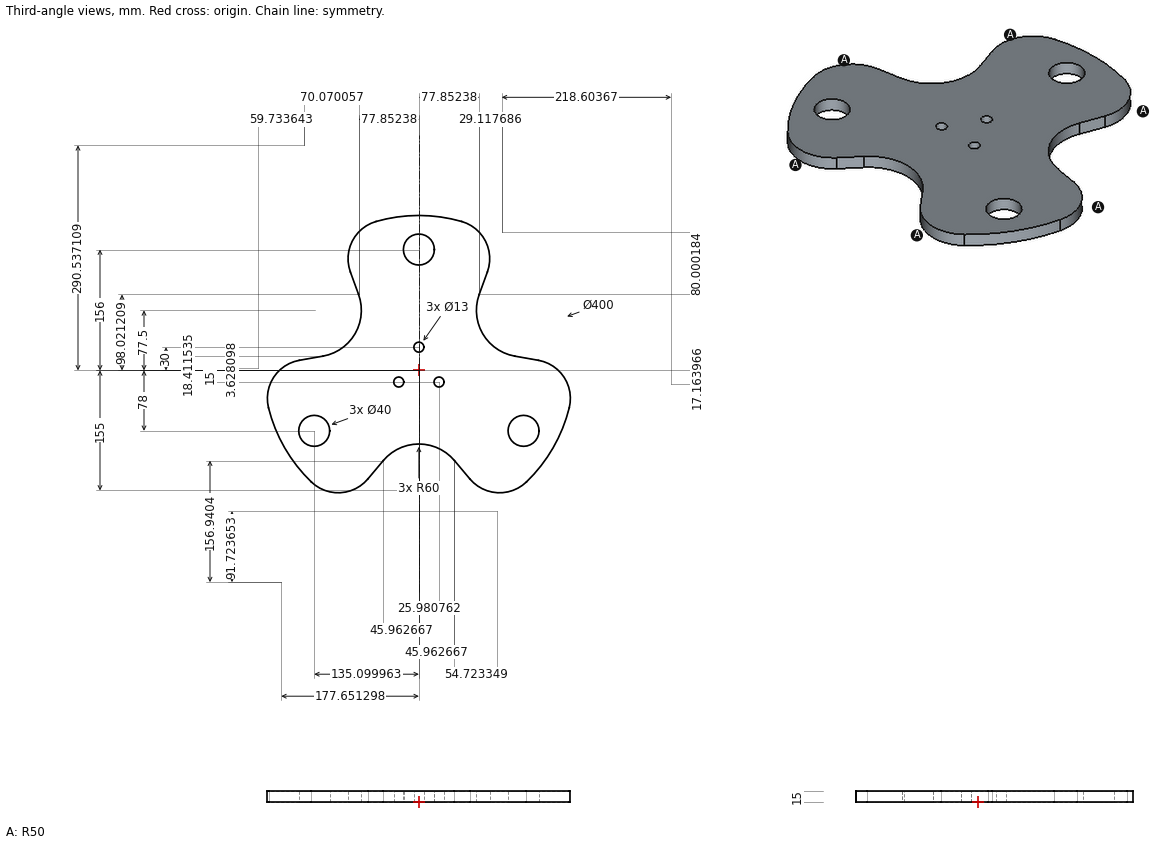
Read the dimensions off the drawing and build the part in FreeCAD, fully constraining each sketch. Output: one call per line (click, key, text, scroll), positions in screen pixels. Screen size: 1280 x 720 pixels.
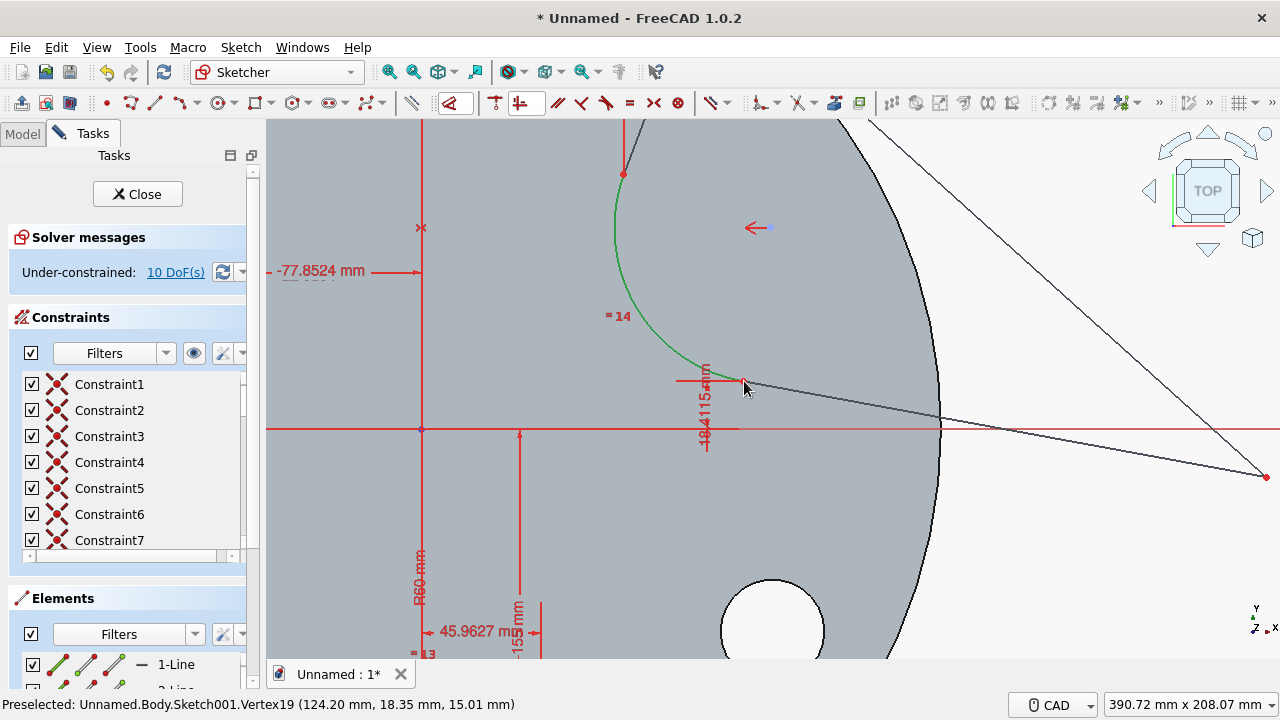
scroll(747, 383, down, 7)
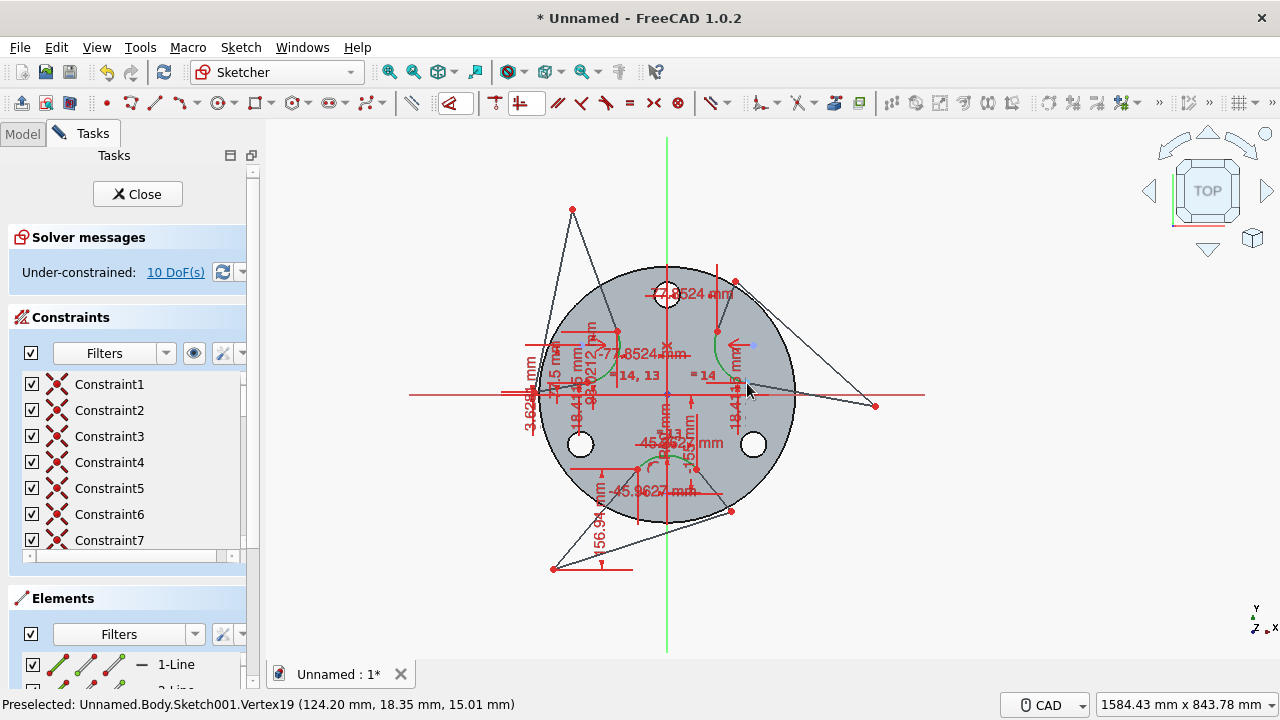
scroll(875, 407, up, 7)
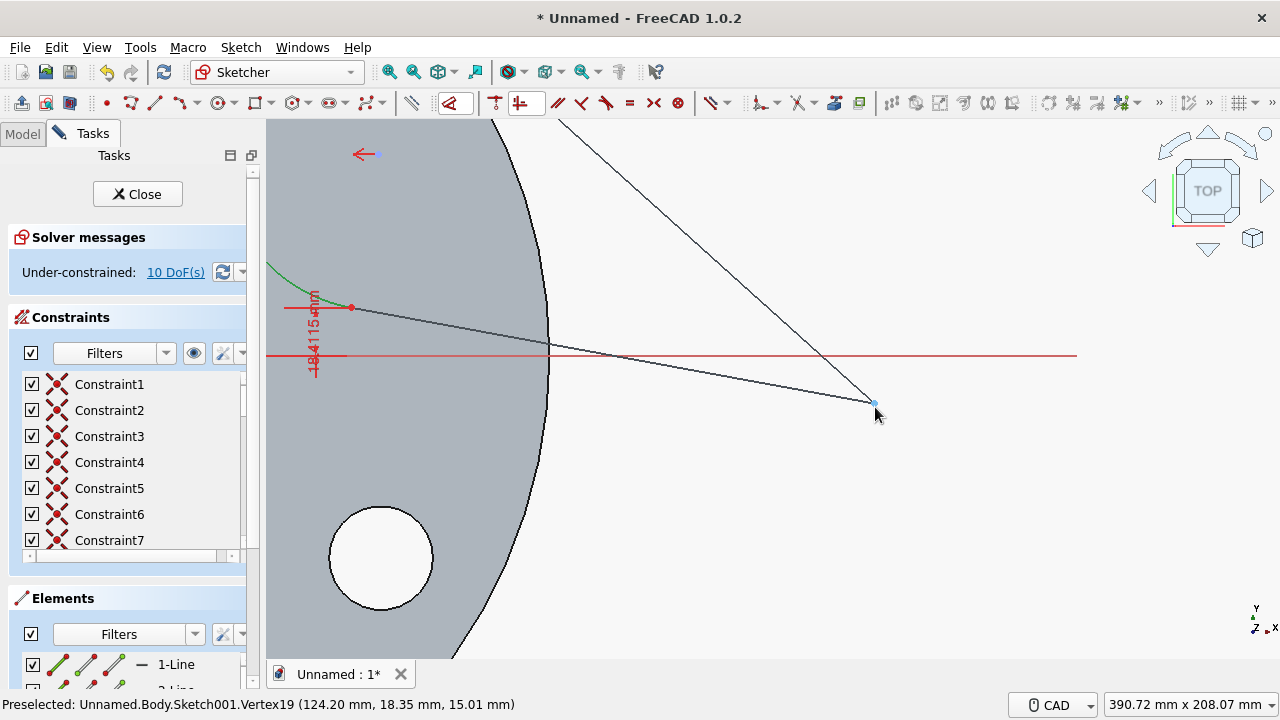
click(875, 404)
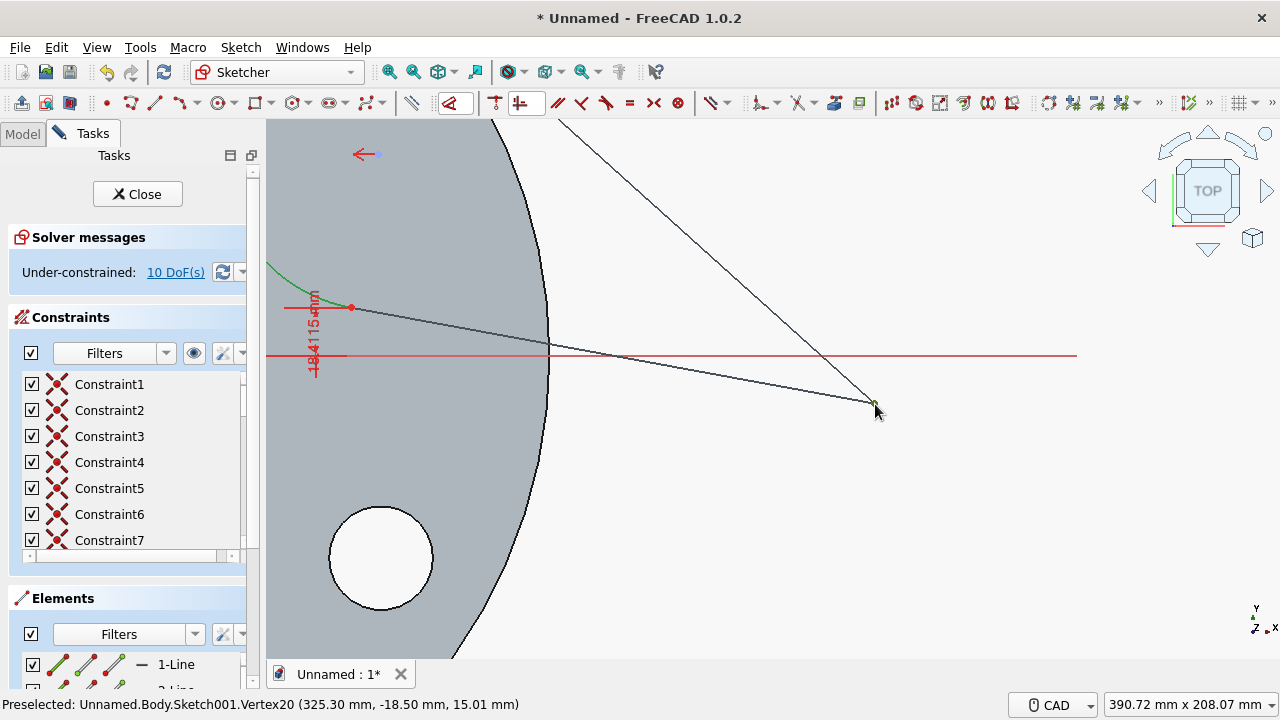
key(i)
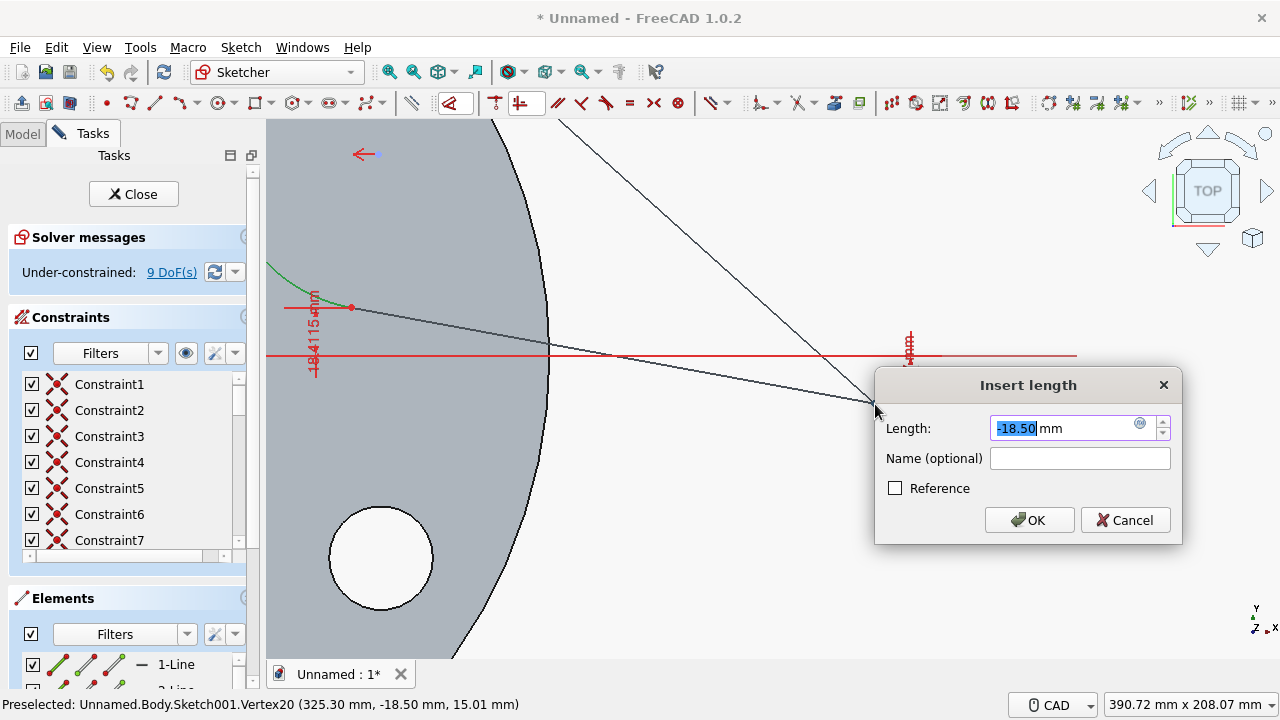
text(-17.163966)
key(Return)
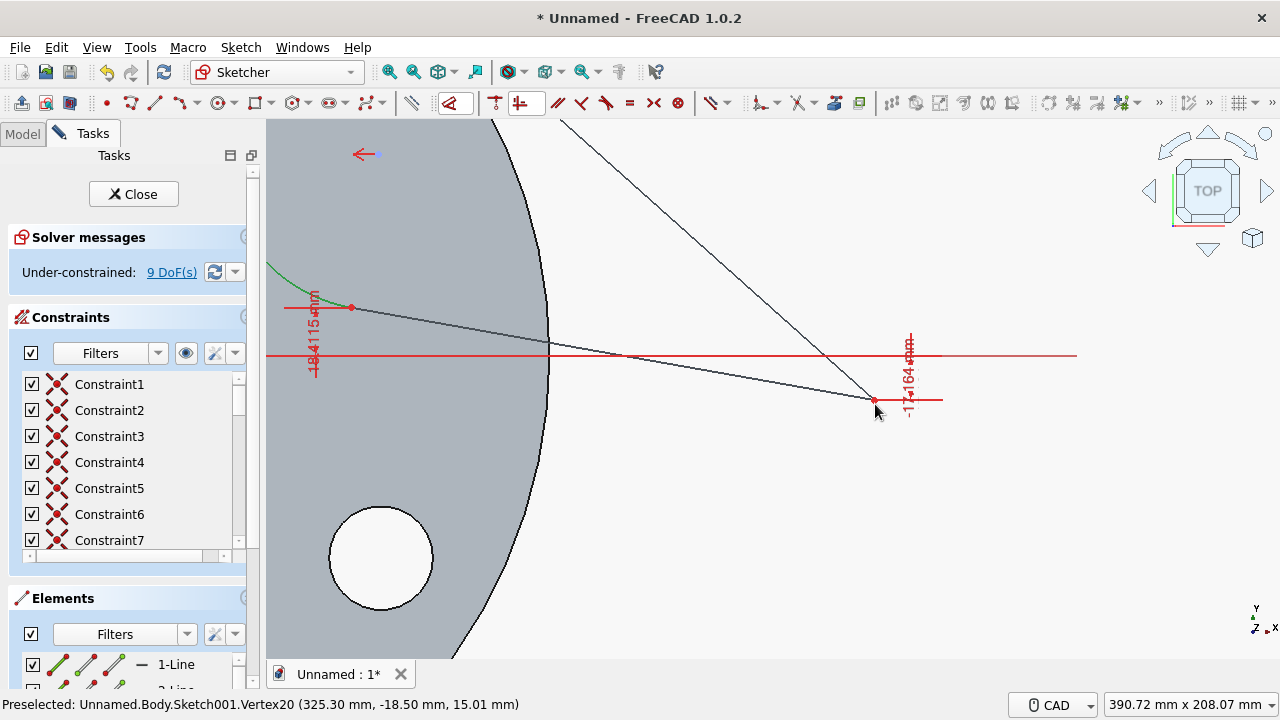
scroll(875, 407, down, 7)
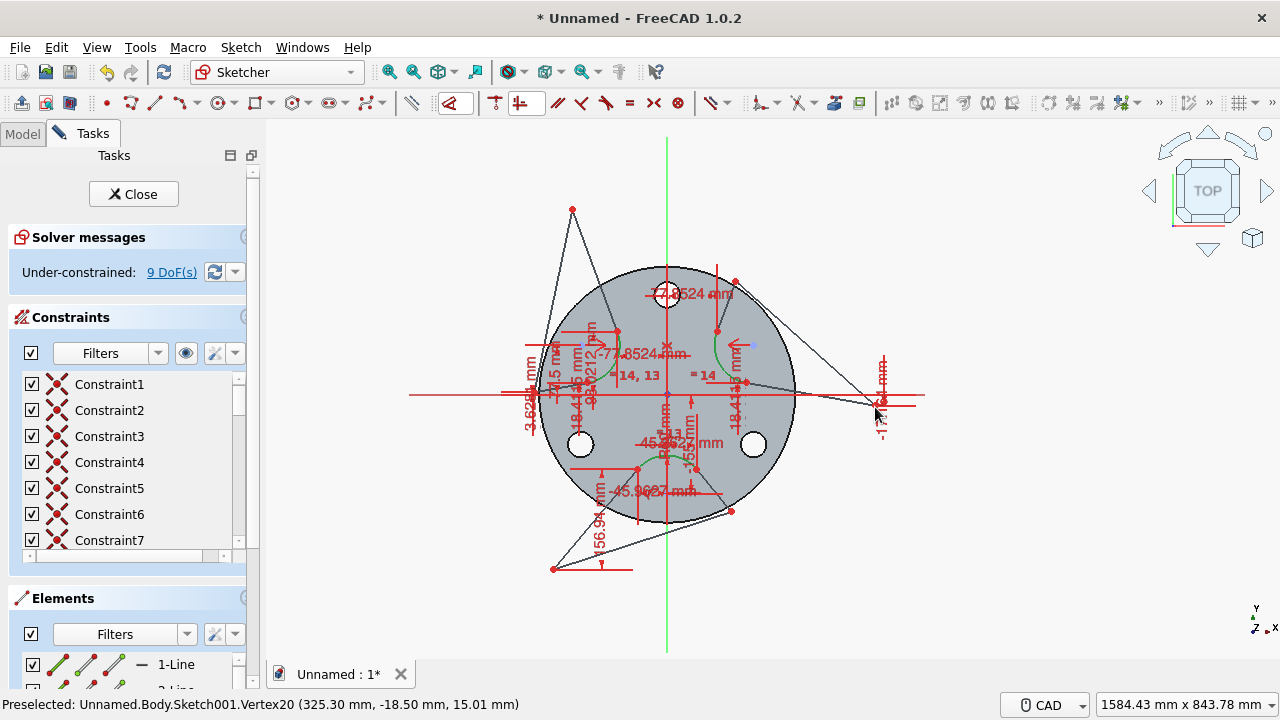
click(678, 529)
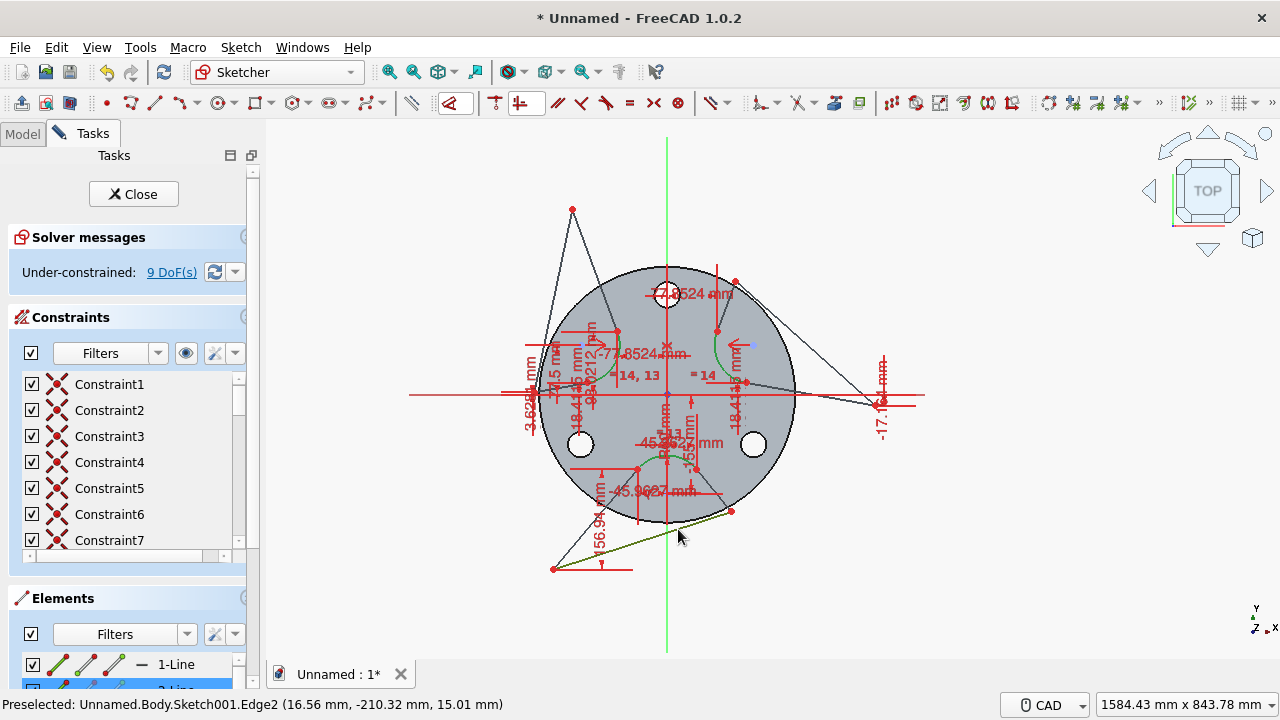
click(468, 104)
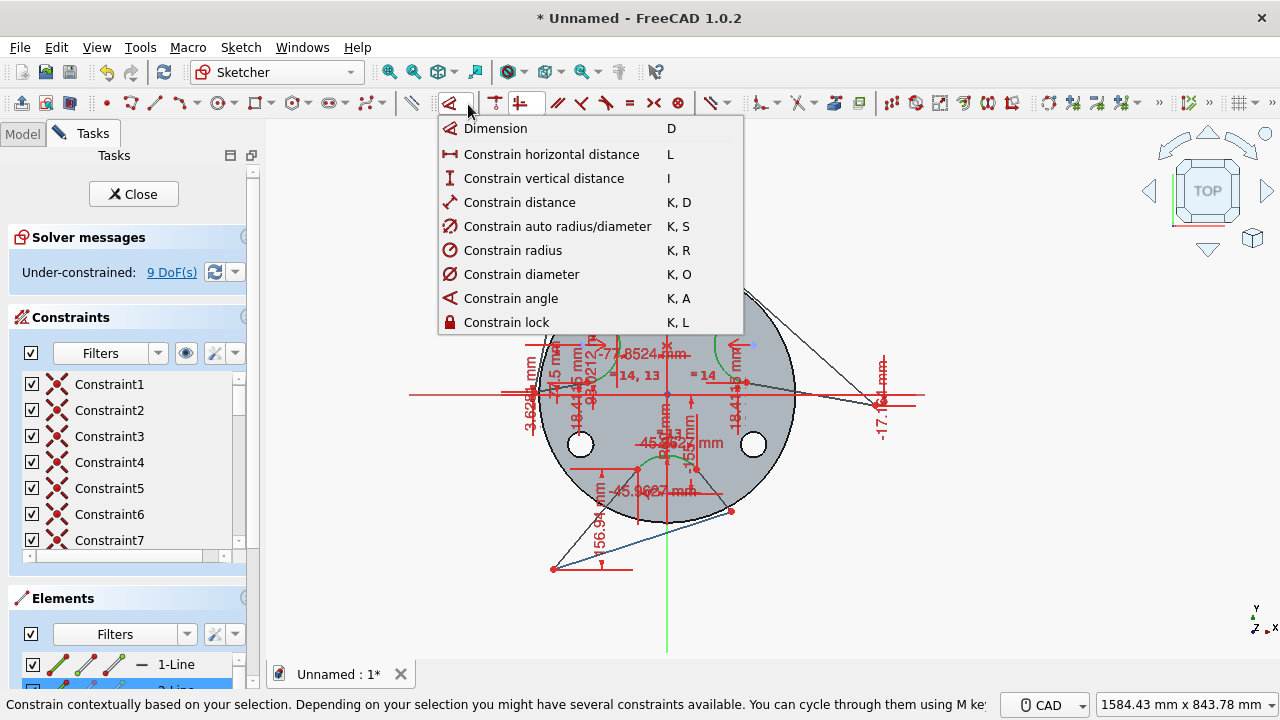
click(591, 178)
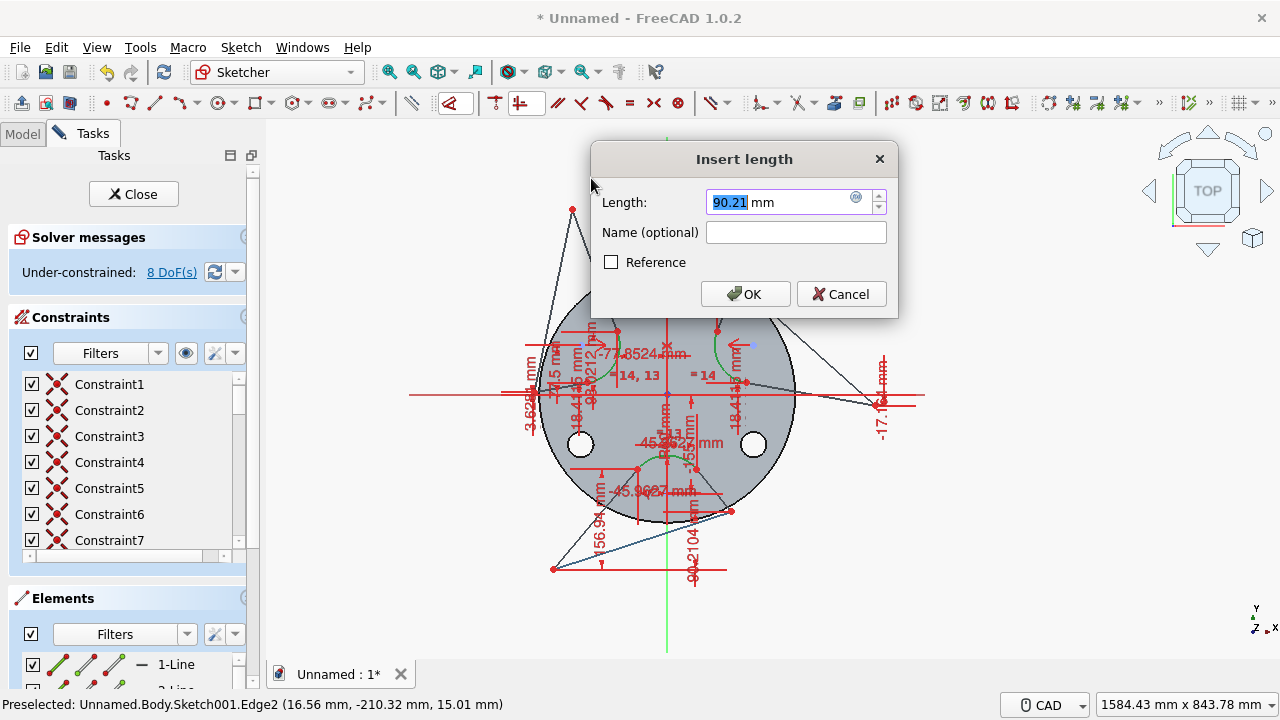
text(91.723653)
key(Return)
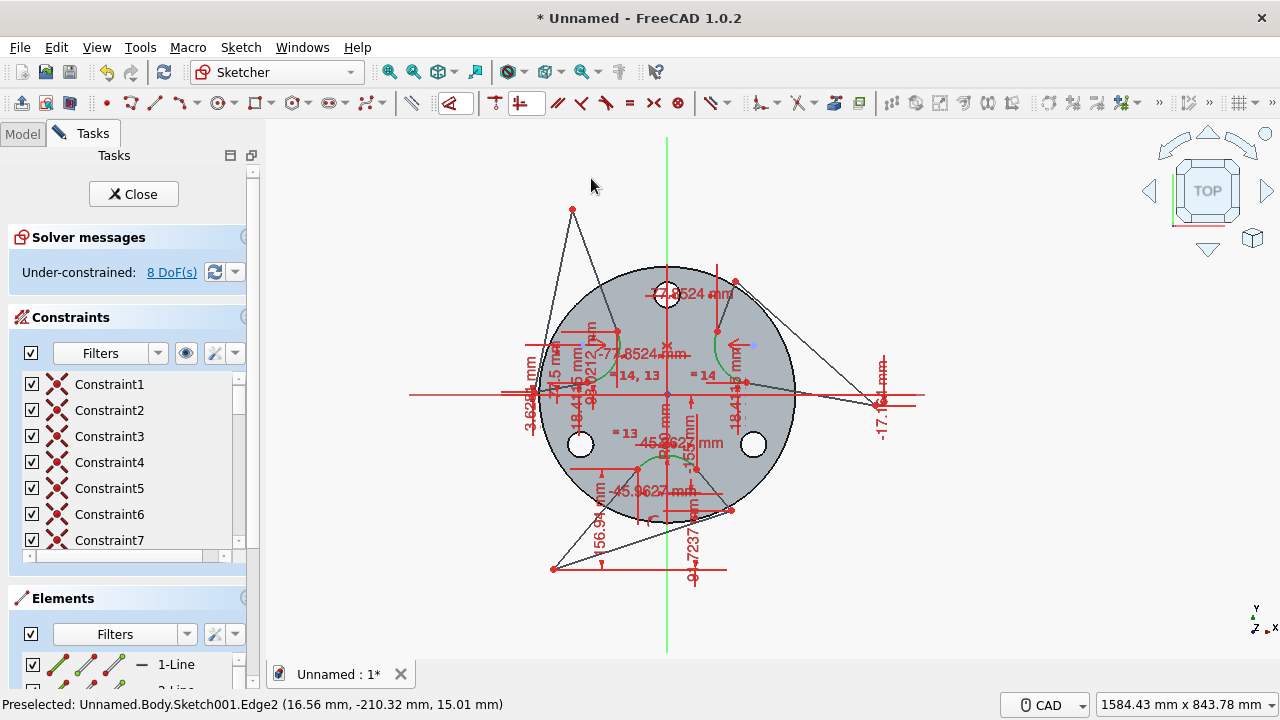
click(721, 498)